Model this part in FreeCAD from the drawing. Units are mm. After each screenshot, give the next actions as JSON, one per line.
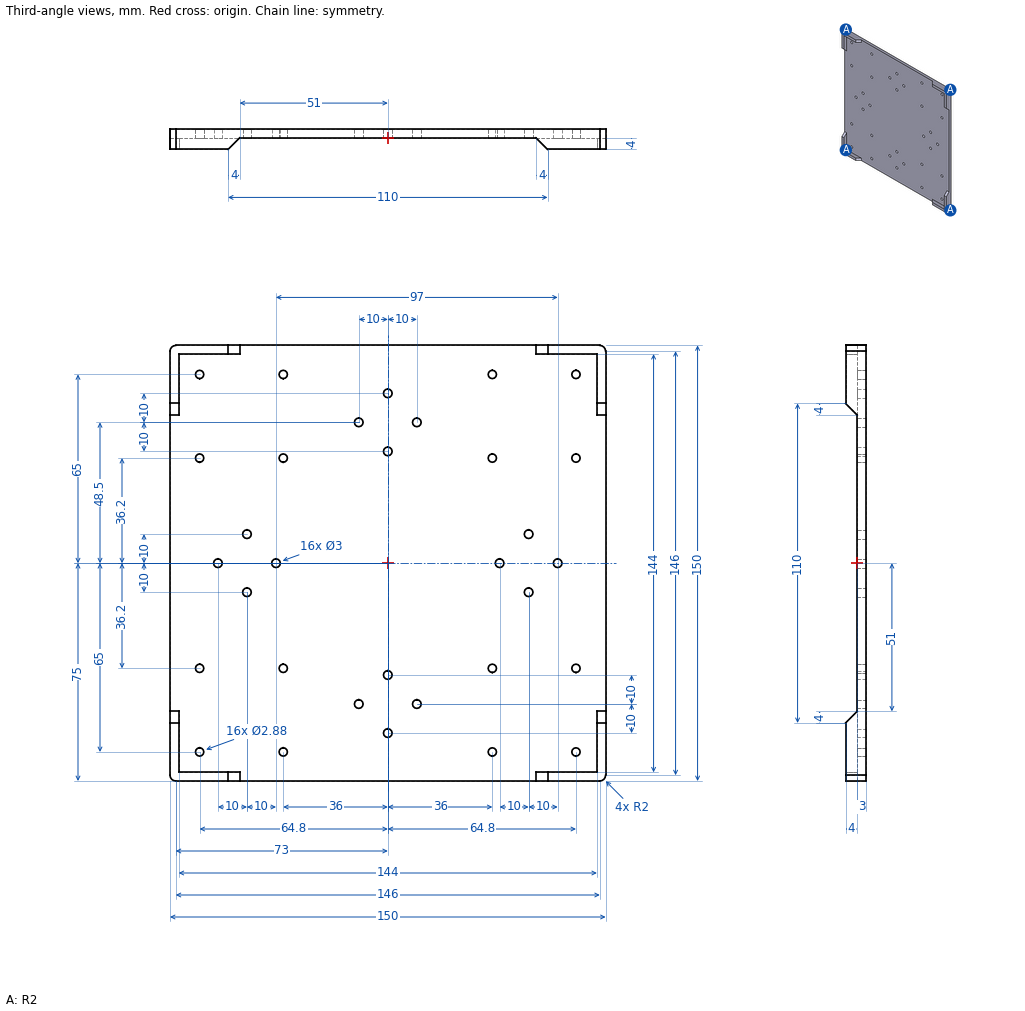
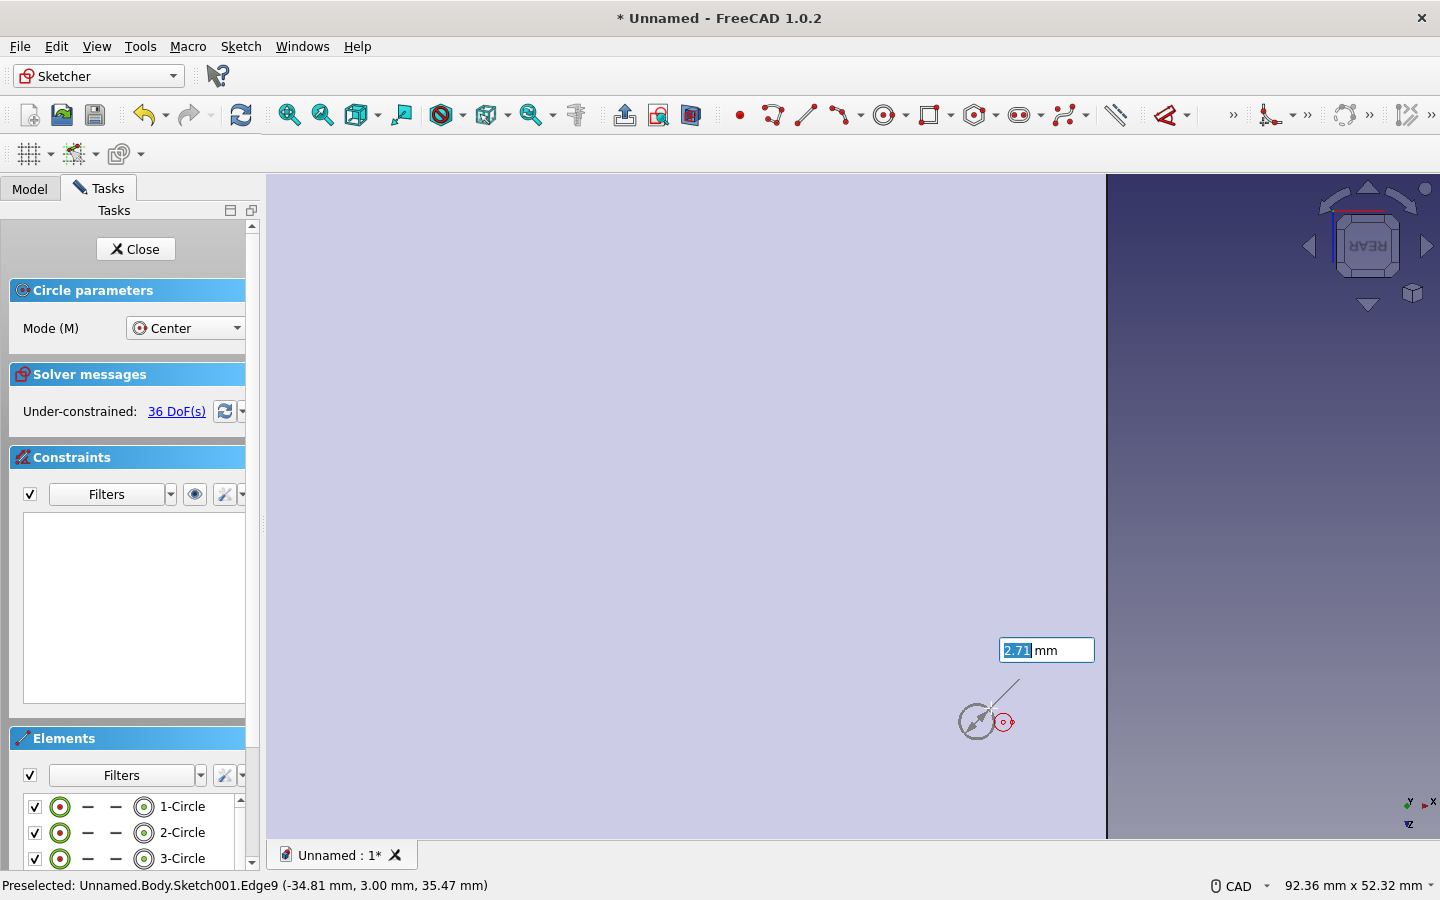
{"action": "left_click", "coordinate": [990, 704]}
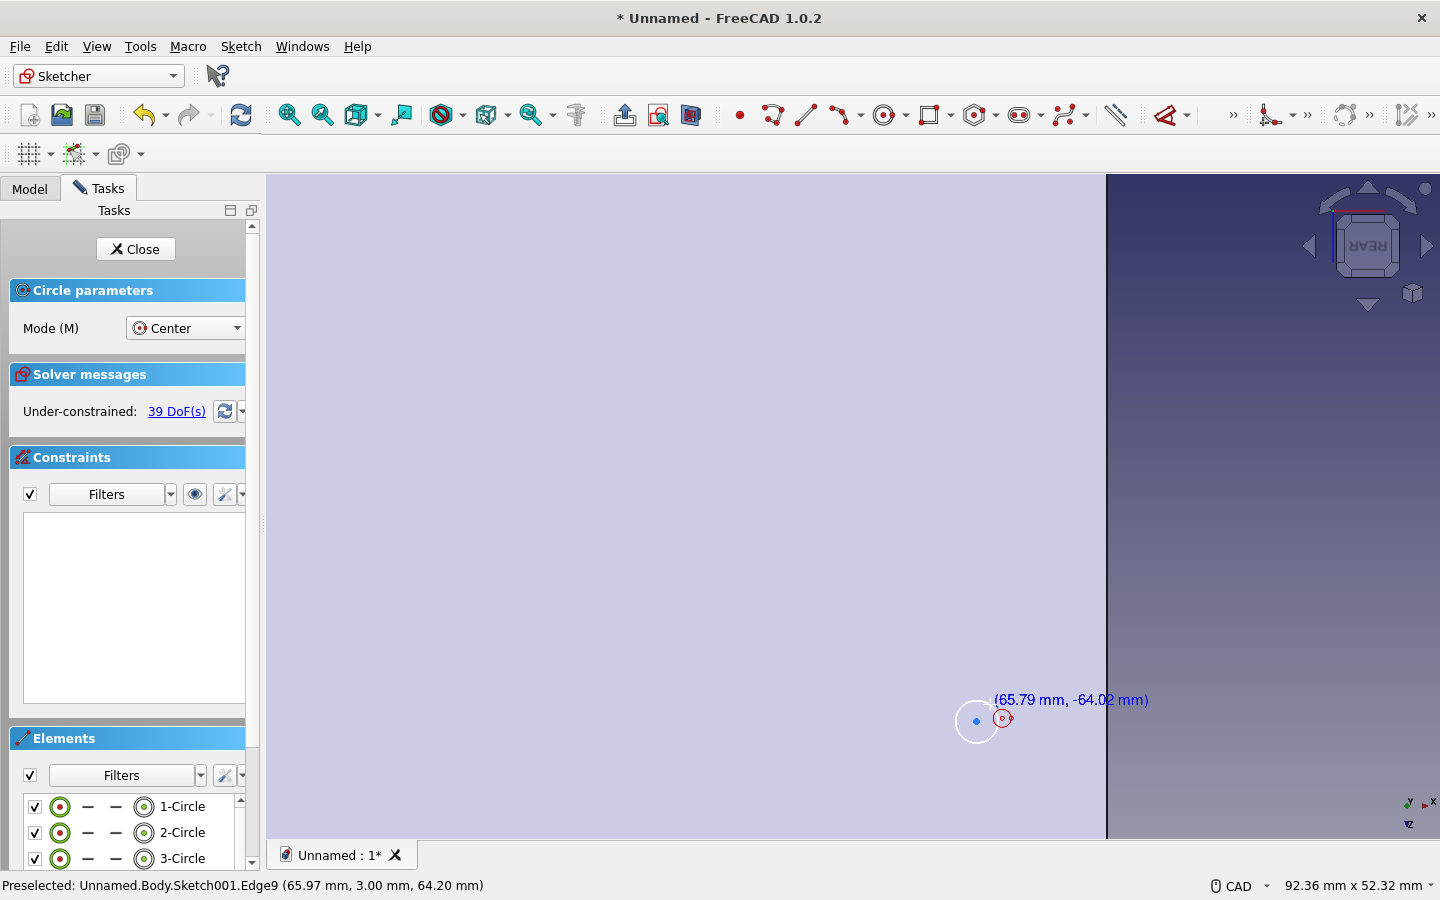
{"action": "scroll", "coordinate": [611, 717], "scroll_direction": "up", "scroll_amount": 2}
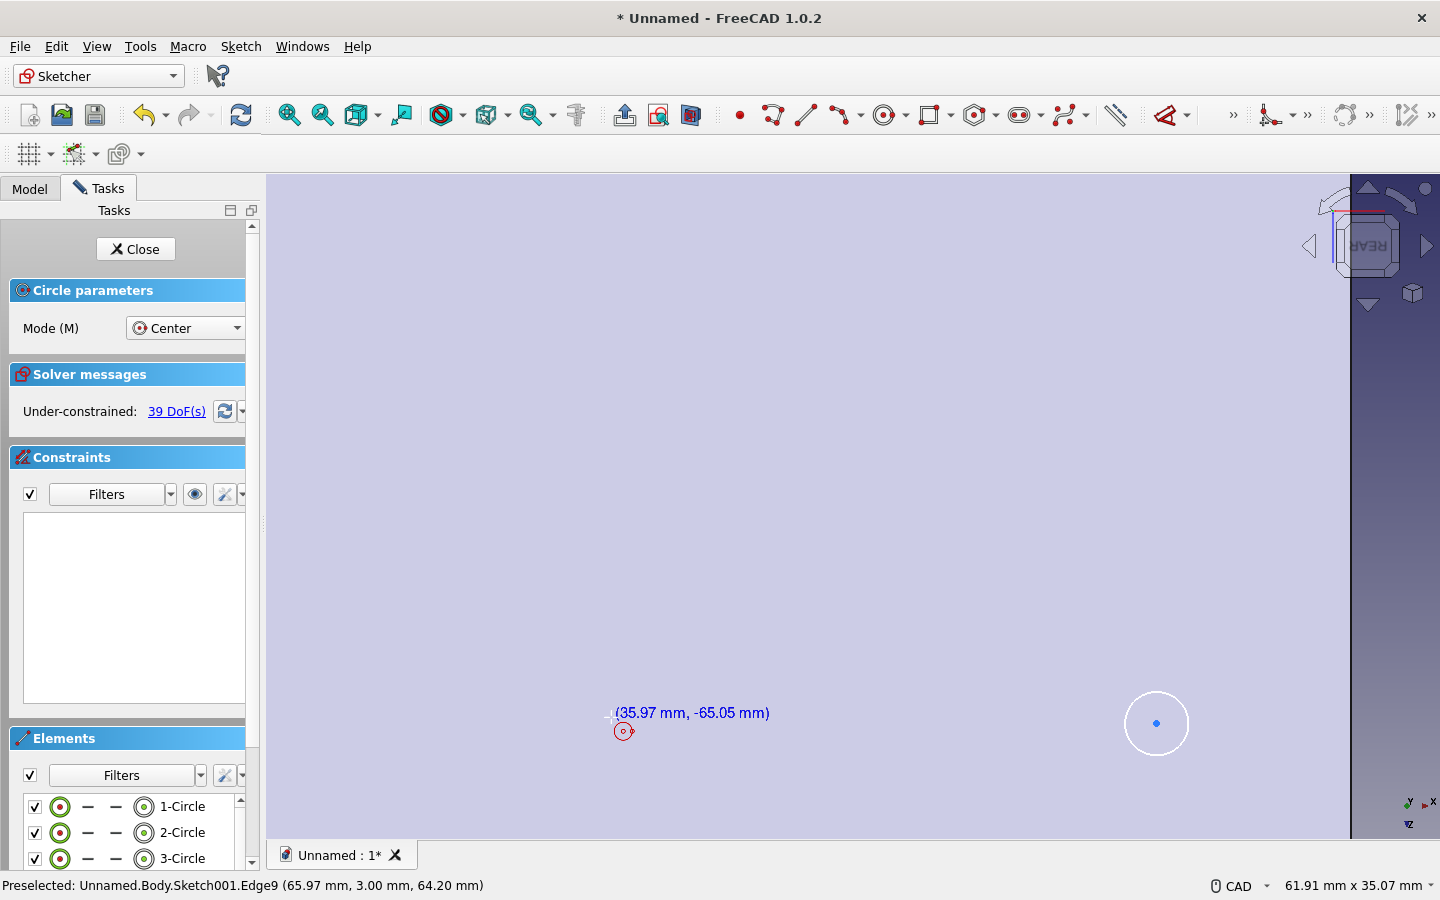
{"action": "scroll", "coordinate": [954, 709], "scroll_direction": "down", "scroll_amount": 9}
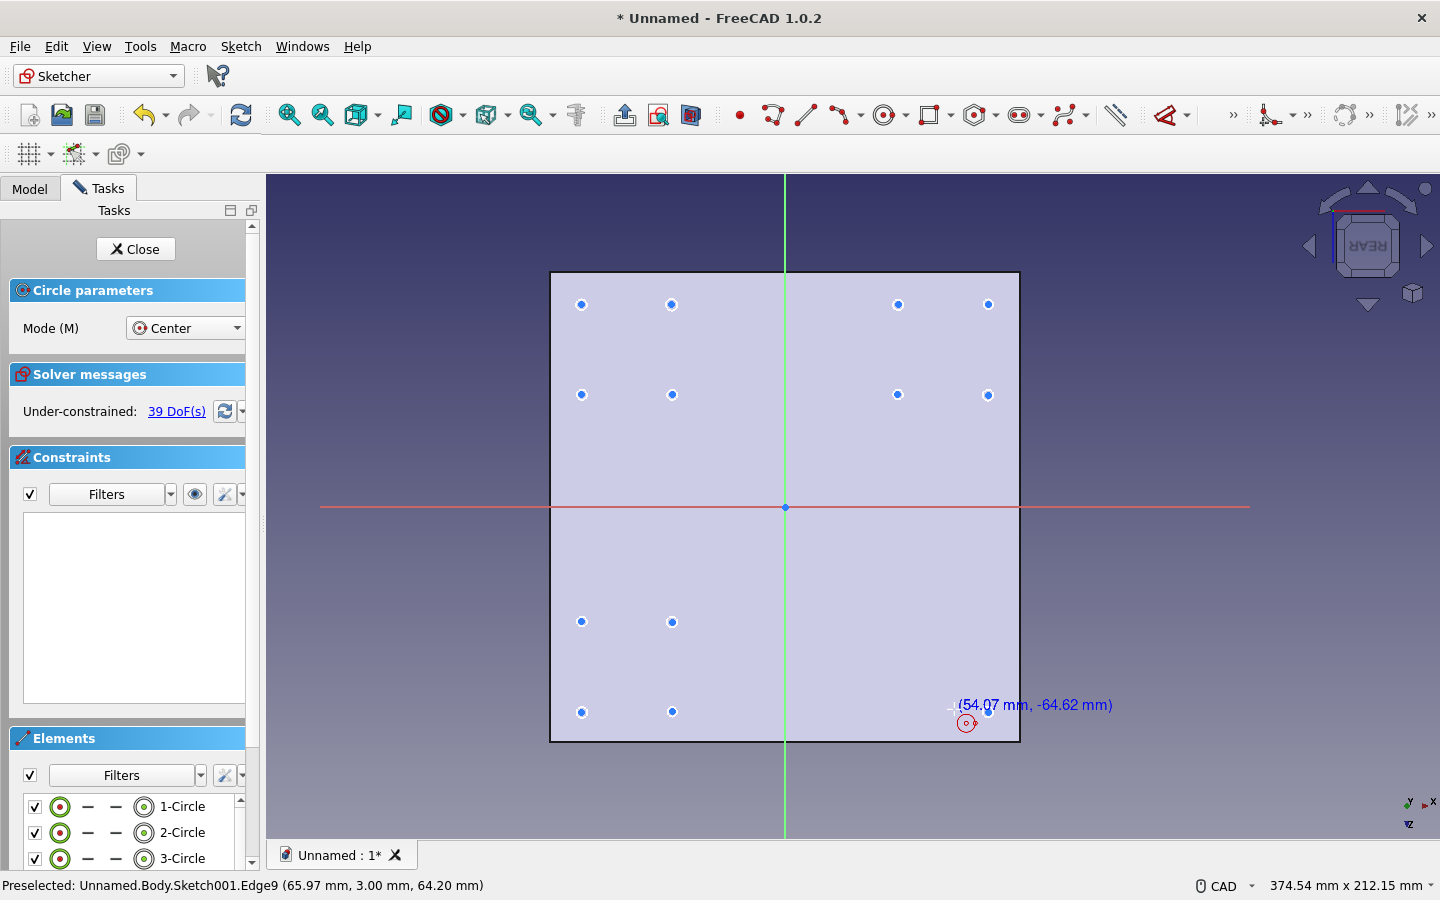
{"action": "left_click", "coordinate": [898, 711]}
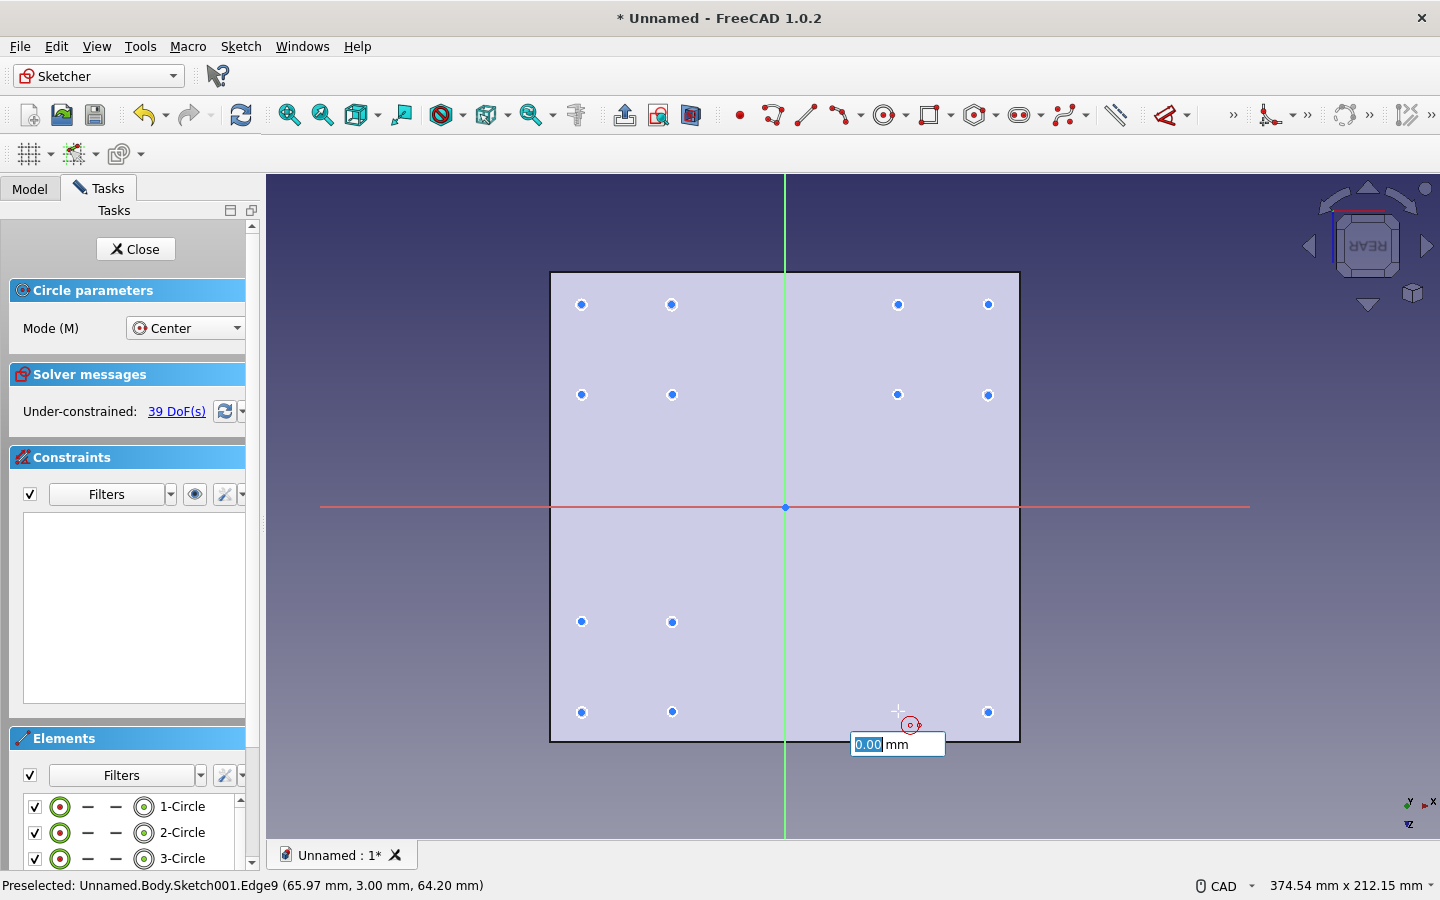
{"action": "scroll", "coordinate": [901, 708], "scroll_direction": "up", "scroll_amount": 7}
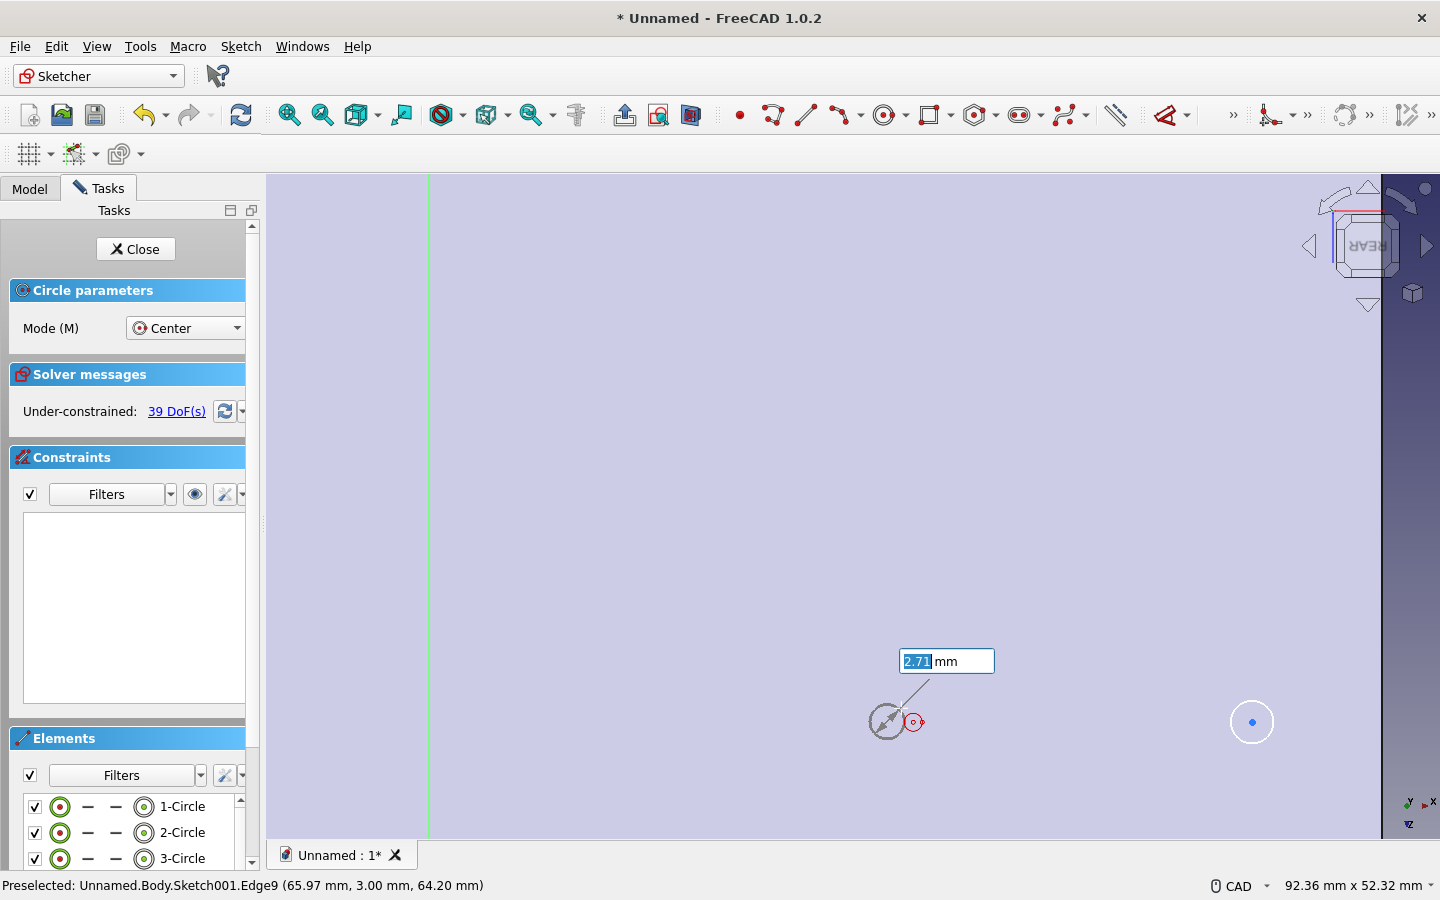
{"action": "left_click", "coordinate": [900, 705]}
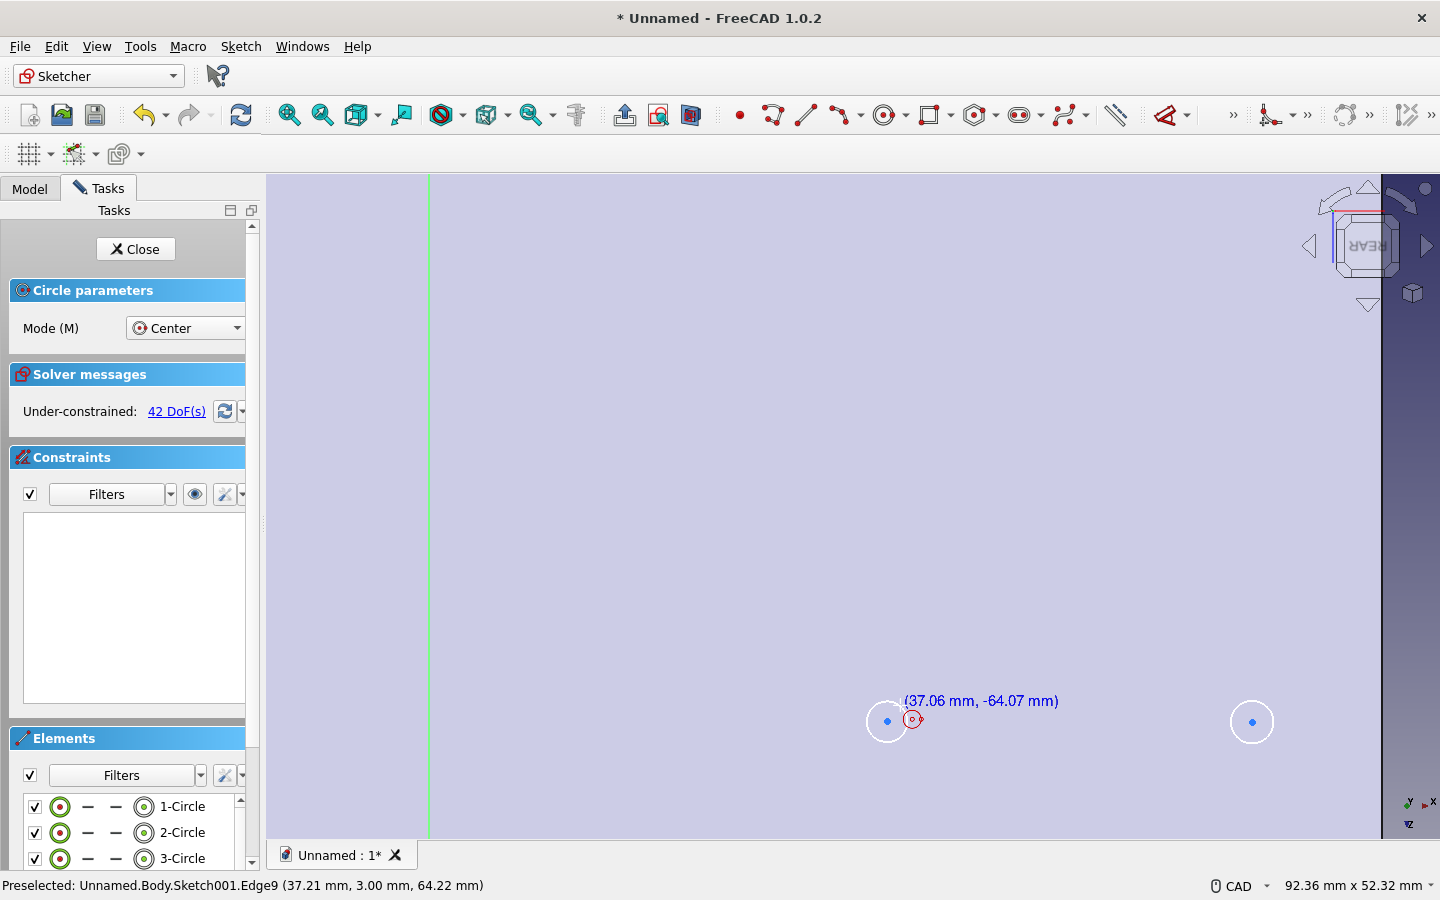
{"action": "scroll", "coordinate": [887, 352], "scroll_direction": "up", "scroll_amount": 2}